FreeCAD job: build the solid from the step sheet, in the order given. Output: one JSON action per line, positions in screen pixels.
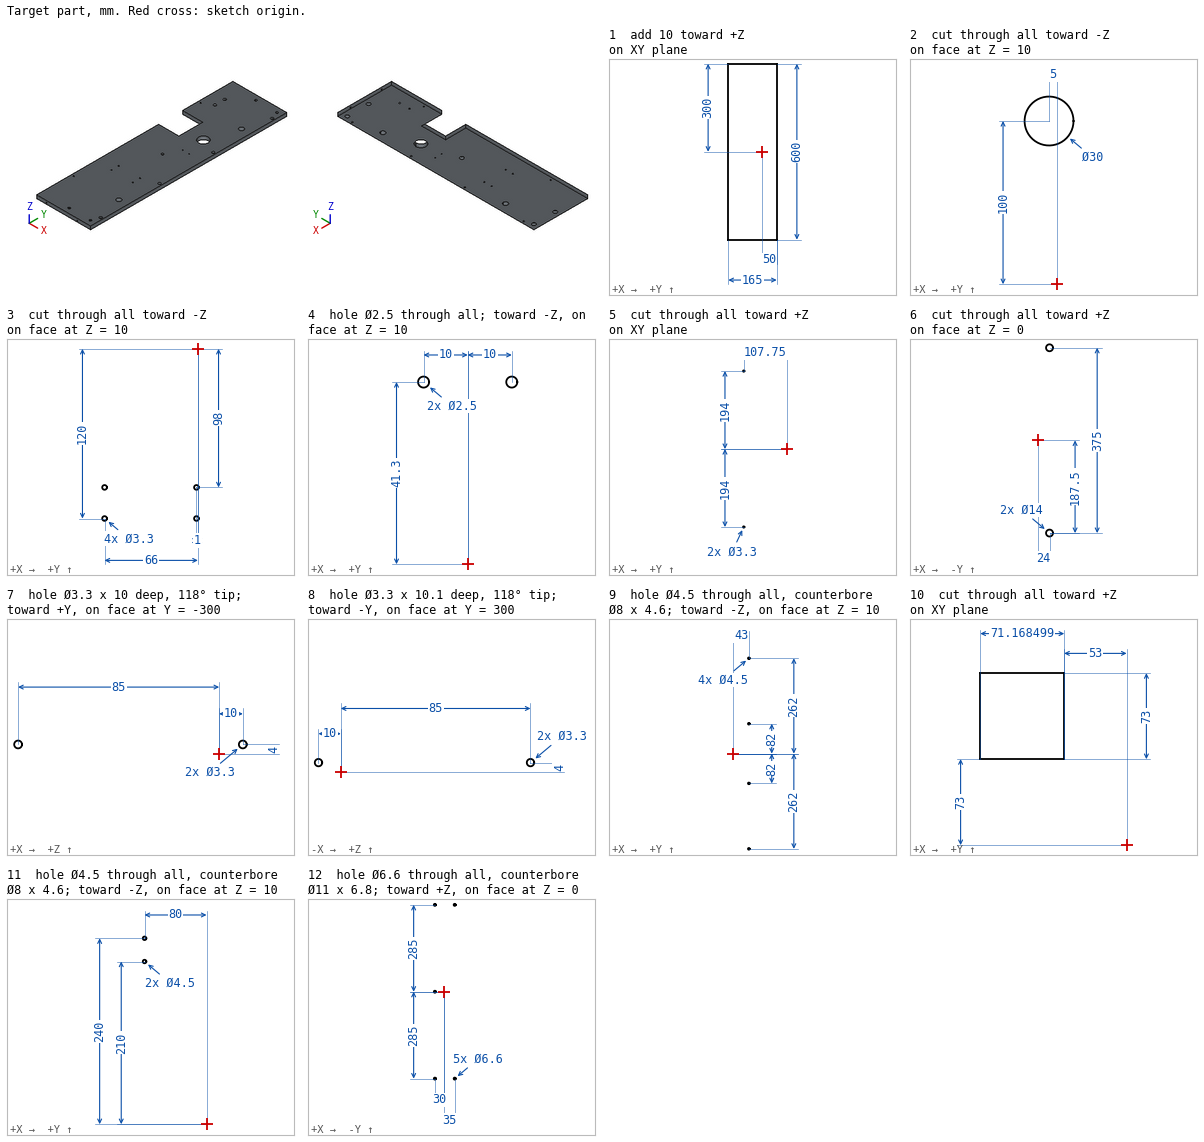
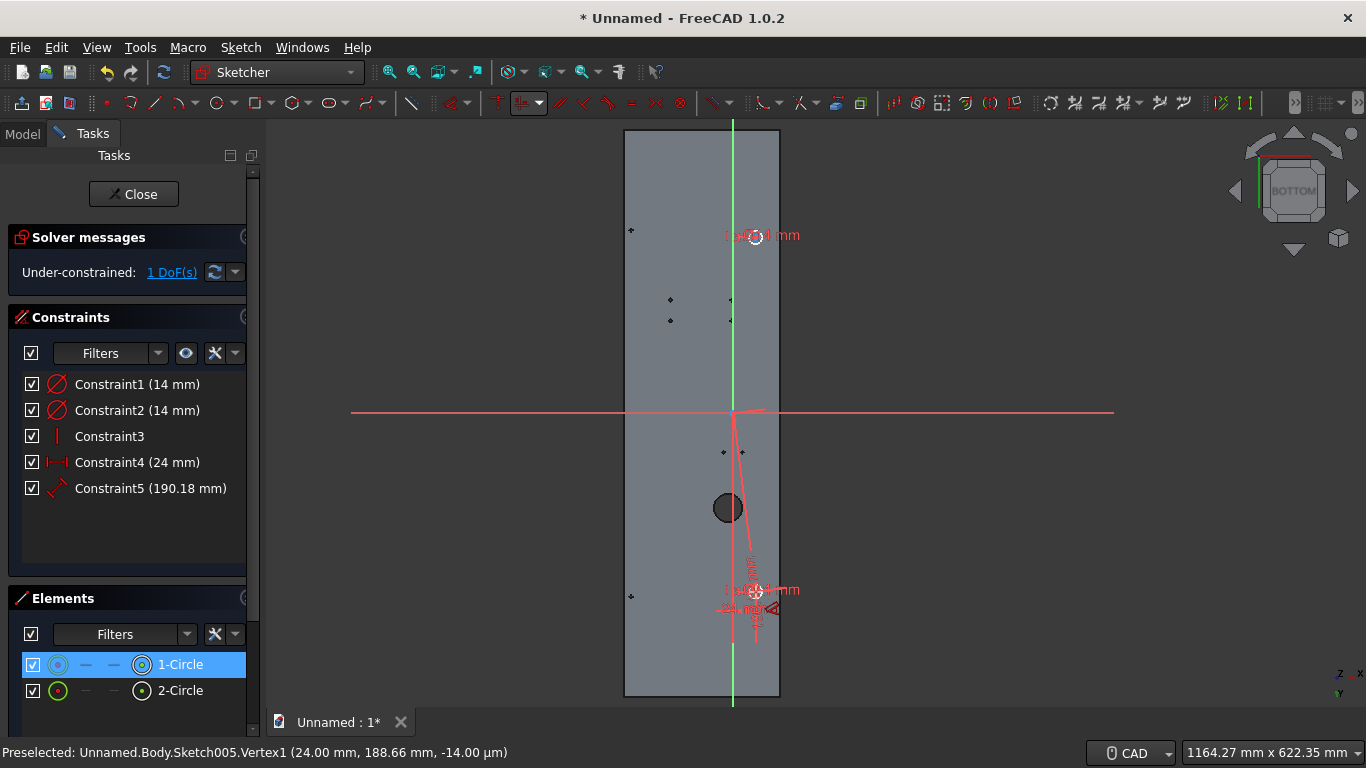
{"action": "left_click", "coordinate": [756, 237]}
{"action": "left_click", "coordinate": [790, 333]}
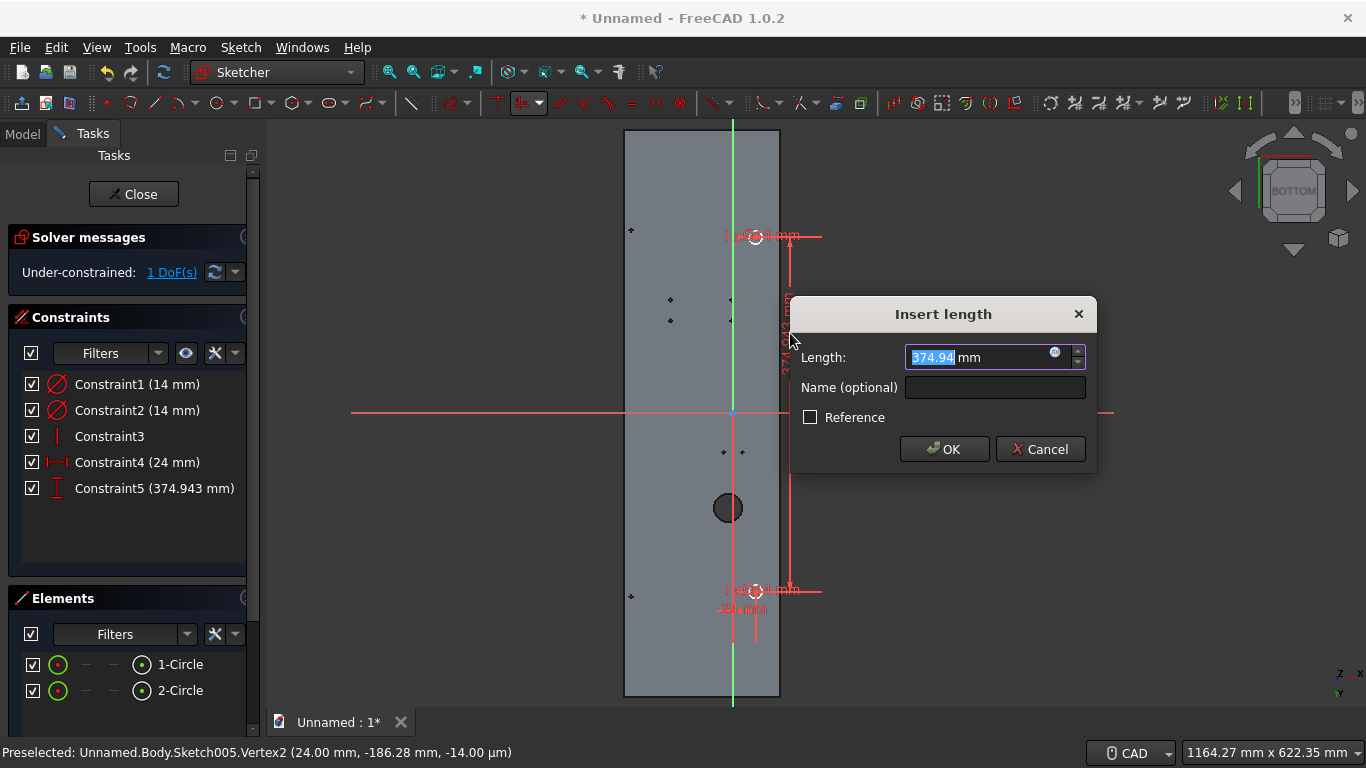
{"action": "type", "text": "375"}
{"action": "key", "text": "Return"}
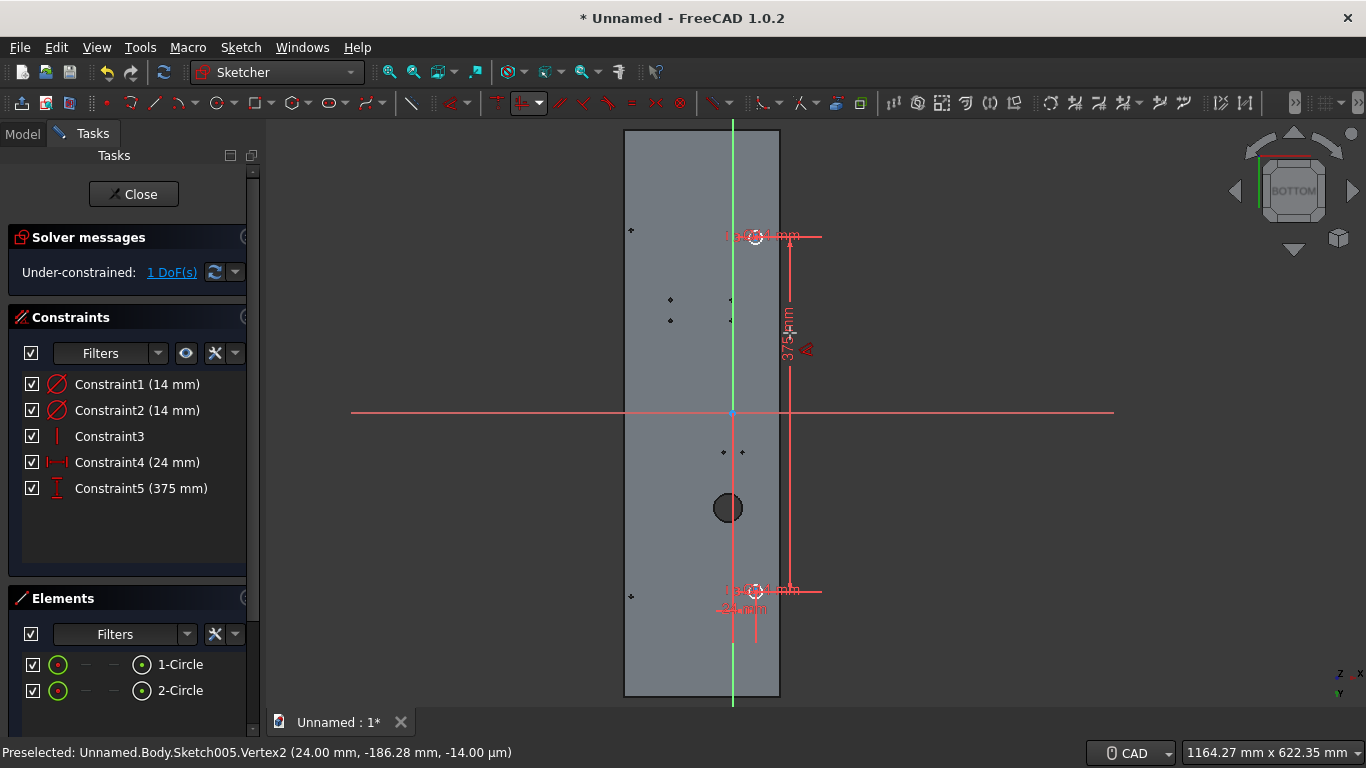
{"action": "left_click", "coordinate": [756, 592]}
{"action": "left_click", "coordinate": [699, 503]}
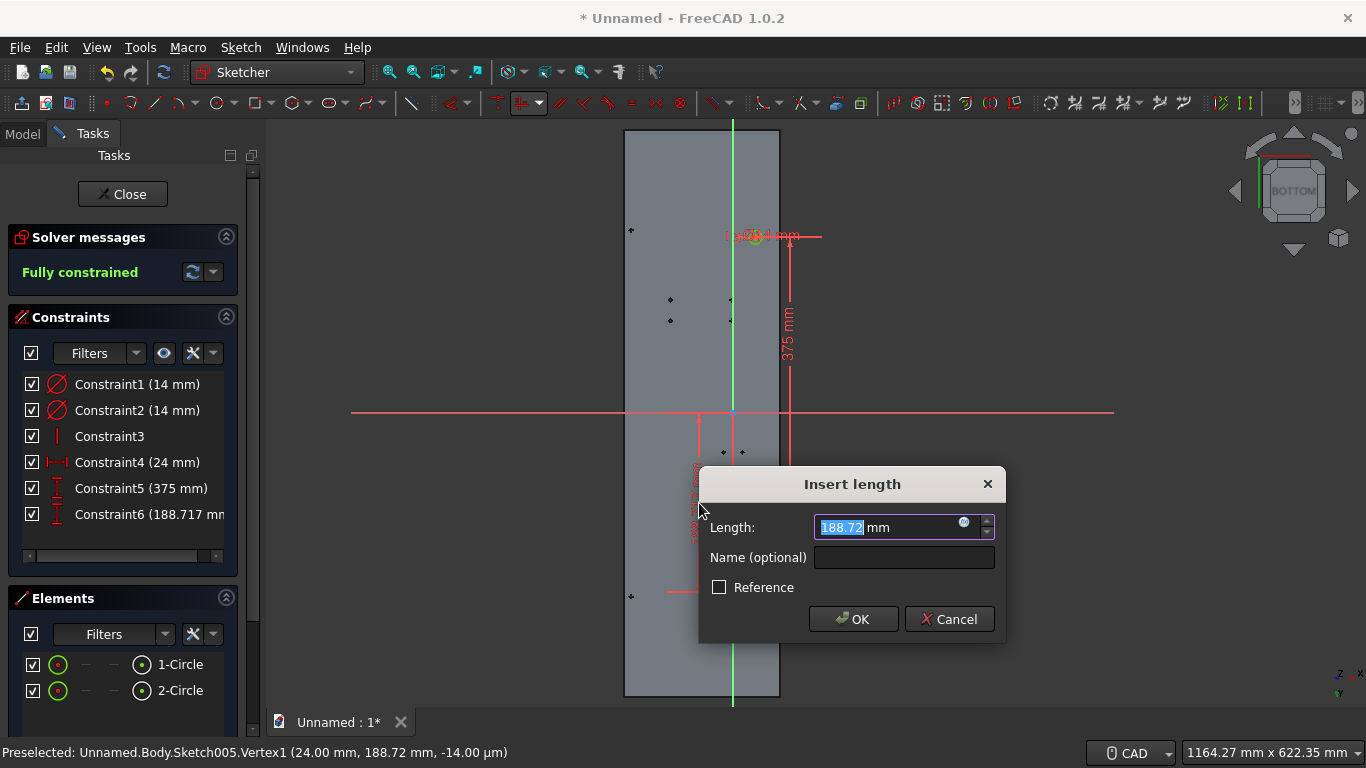
{"action": "type", "text": "187.5"}
{"action": "key", "text": "Return"}
{"action": "key", "text": "Escape"}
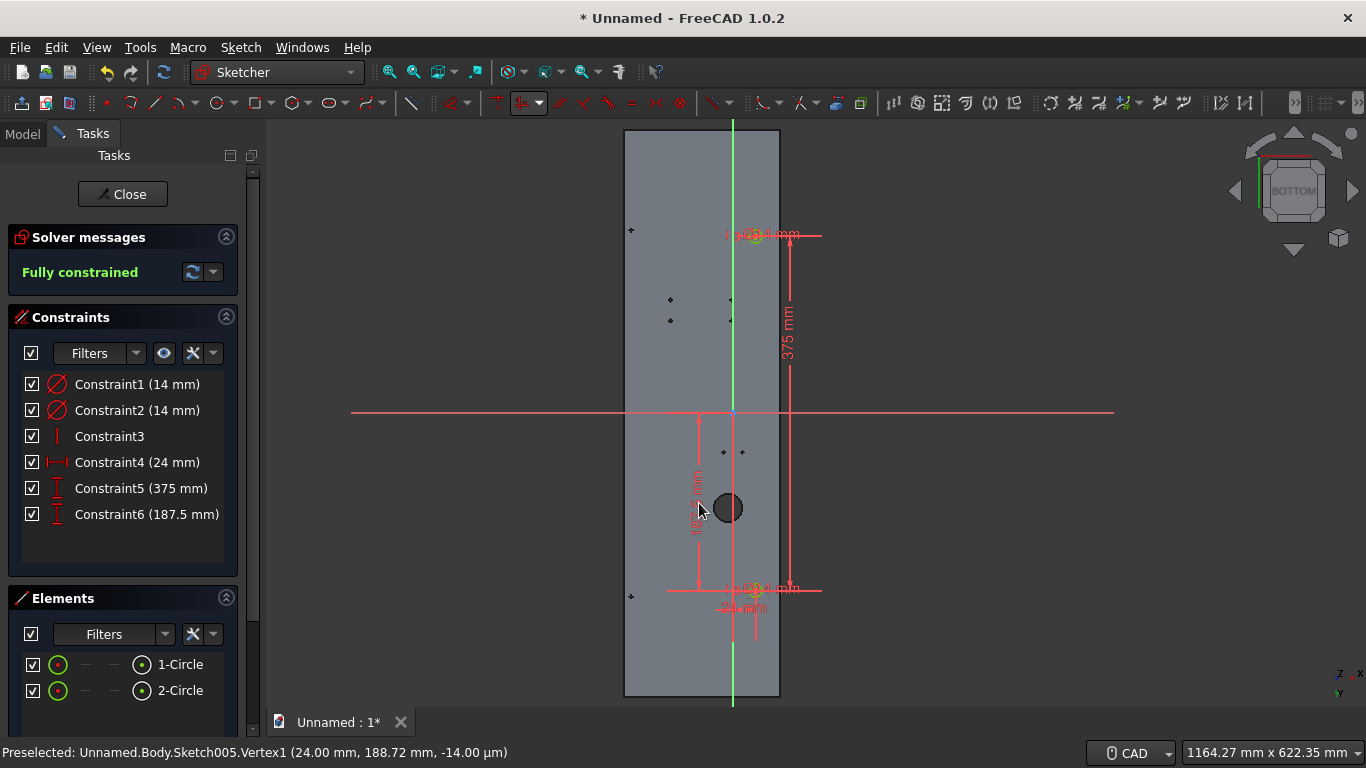
{"action": "left_click", "coordinate": [123, 194]}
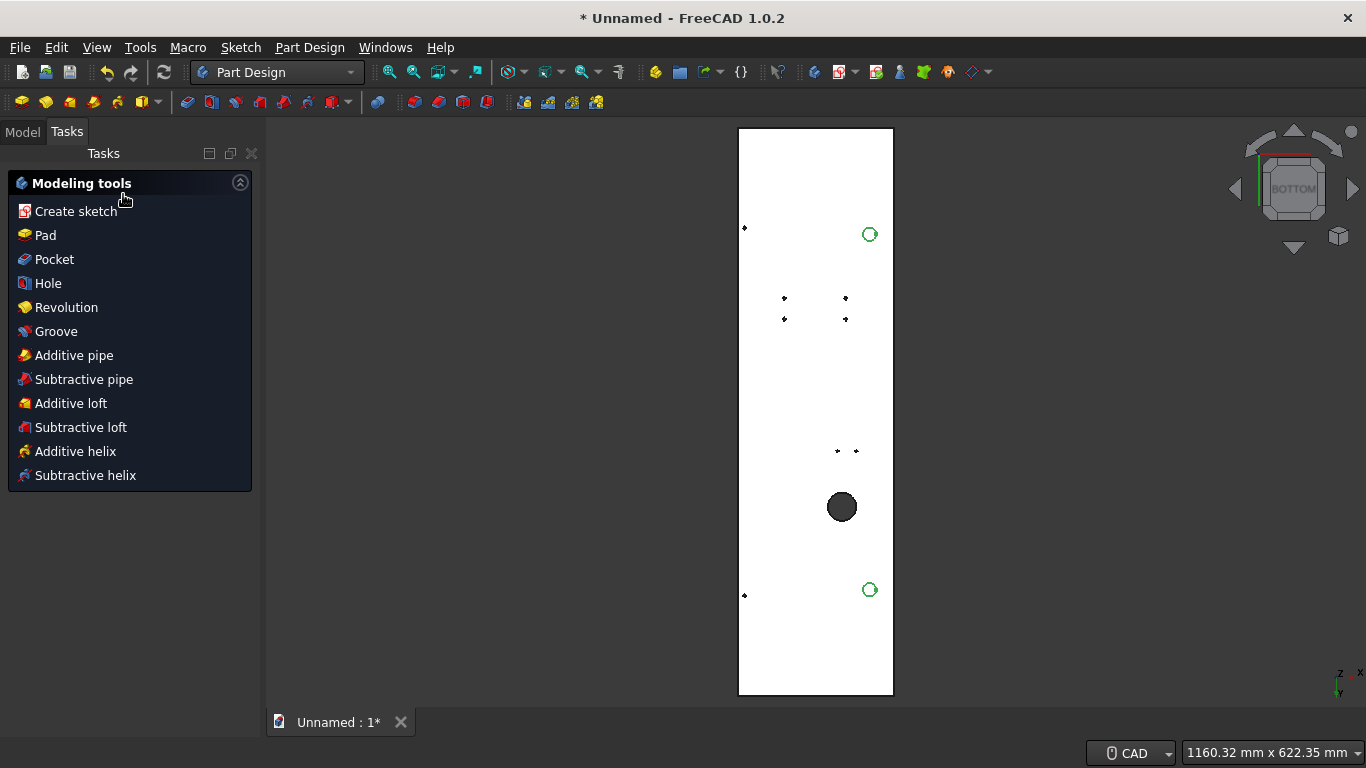
{"action": "left_click", "coordinate": [188, 102]}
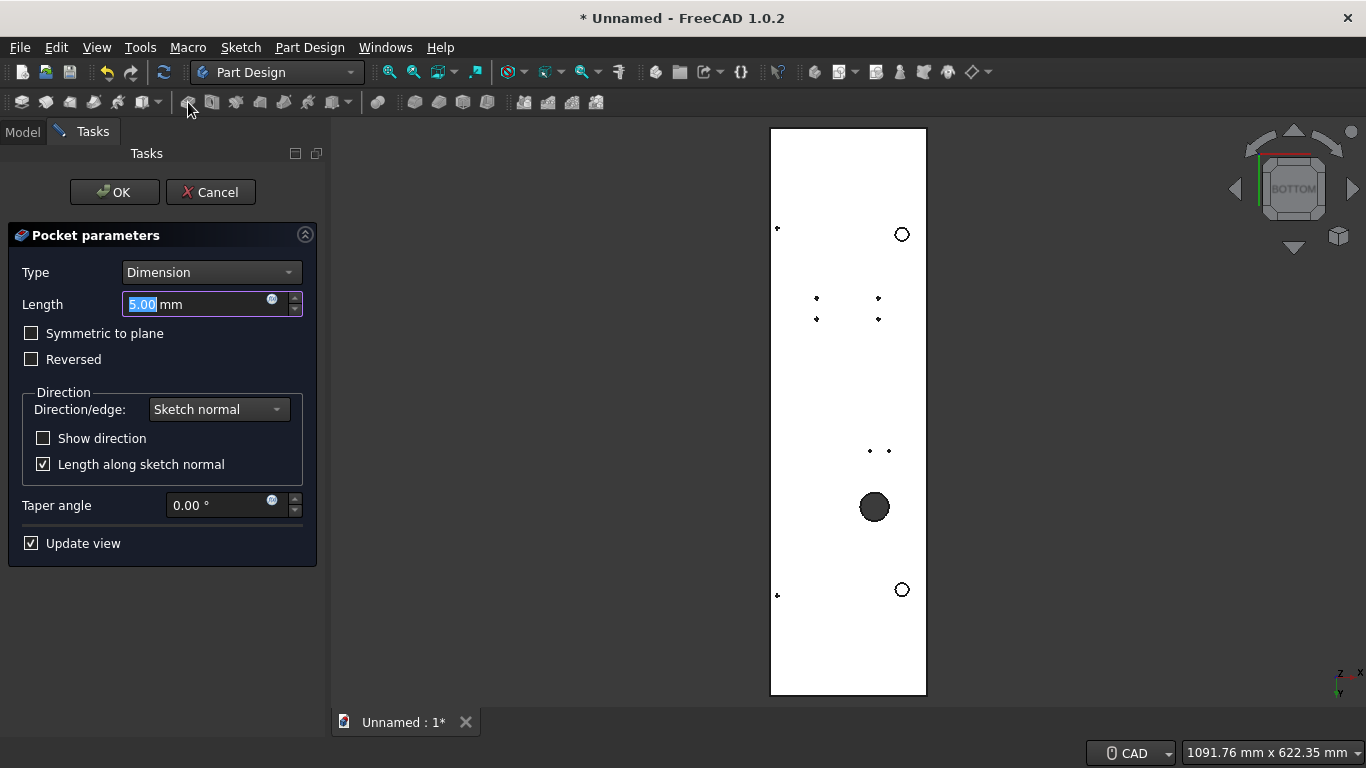
{"action": "left_click", "coordinate": [212, 272]}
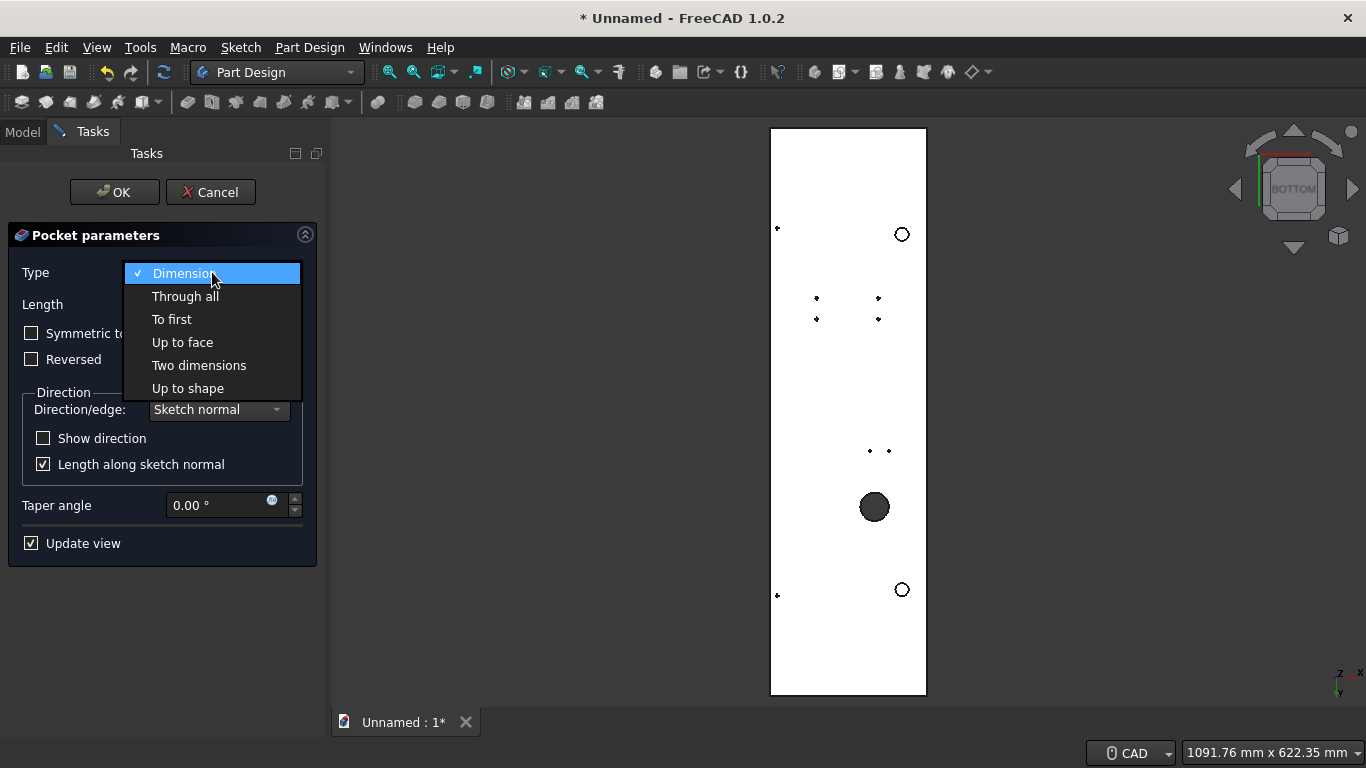
{"action": "left_click", "coordinate": [212, 296]}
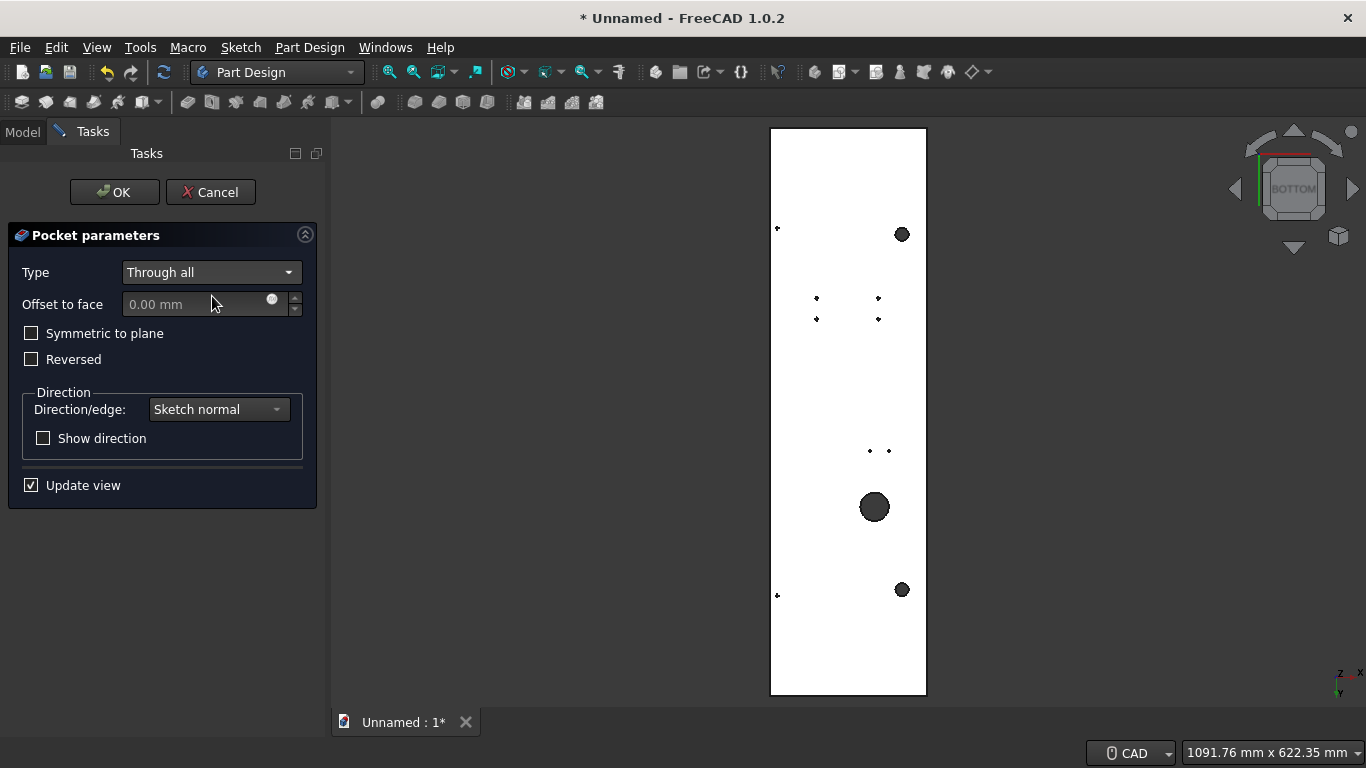
{"action": "left_click", "coordinate": [115, 192]}